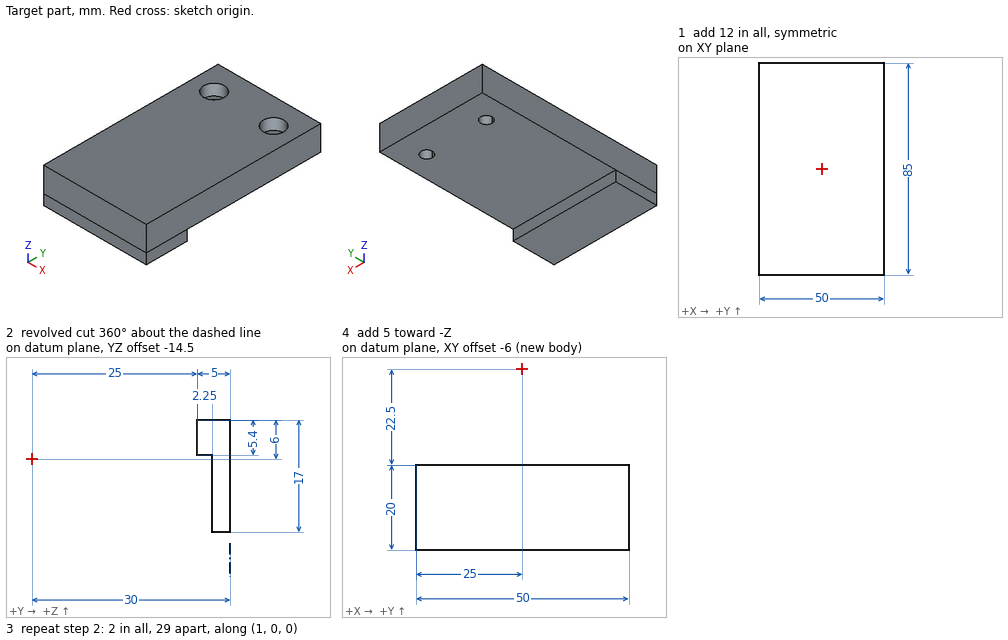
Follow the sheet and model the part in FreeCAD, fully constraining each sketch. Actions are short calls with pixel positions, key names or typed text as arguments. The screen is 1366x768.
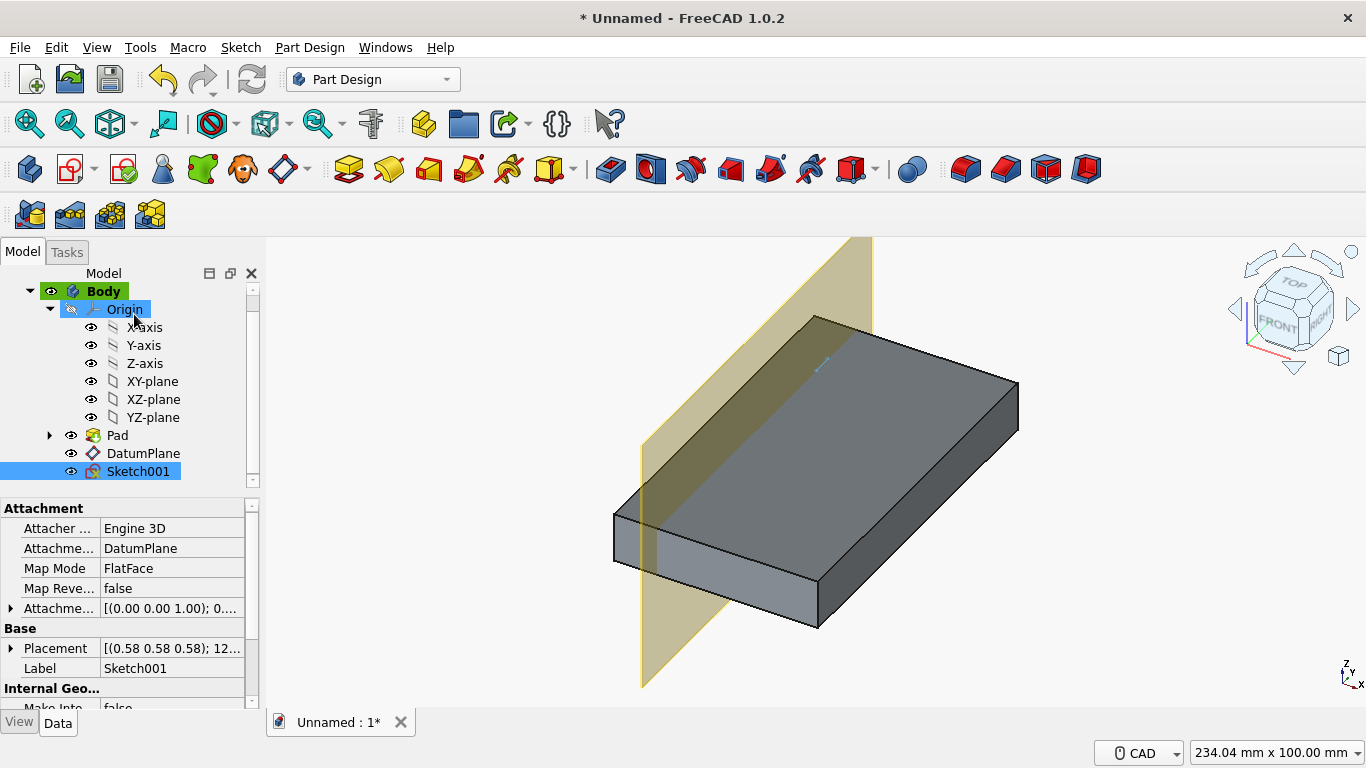
click(692, 170)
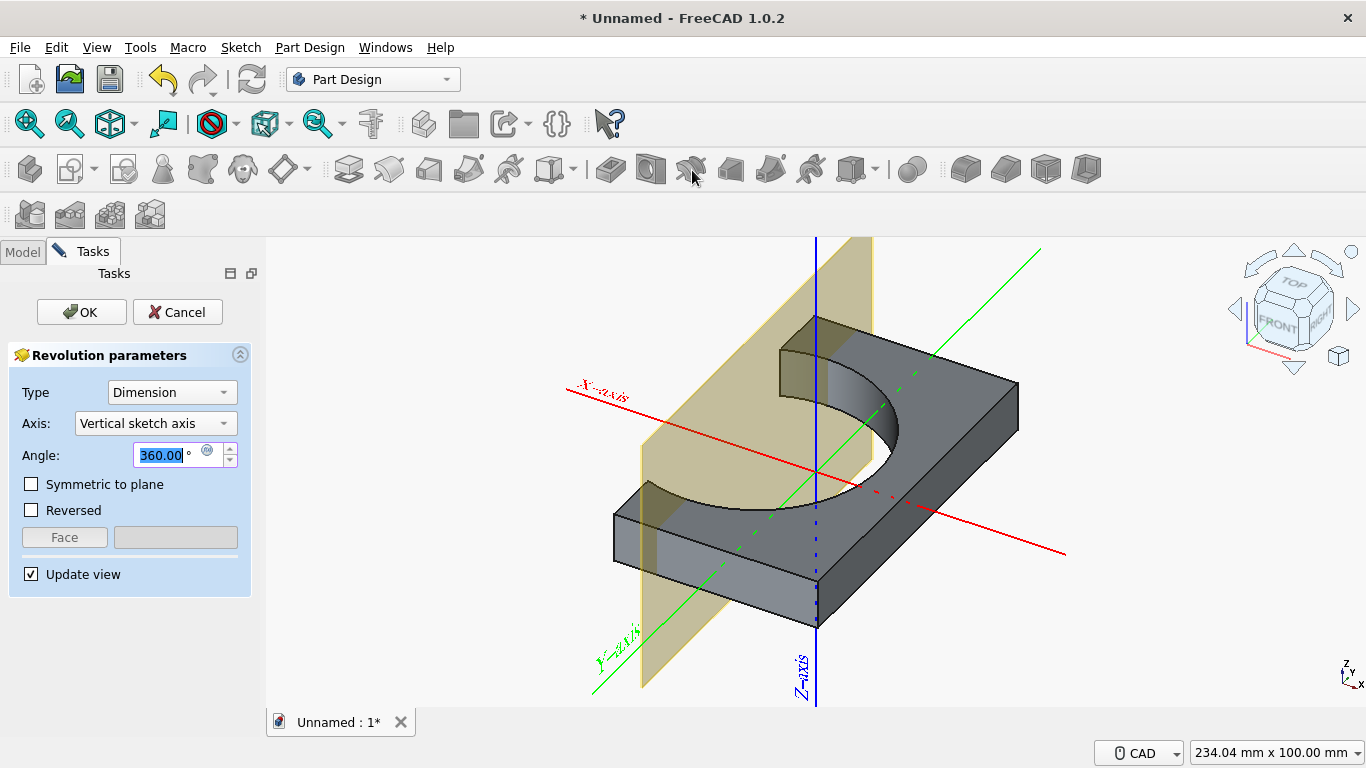
click(156, 424)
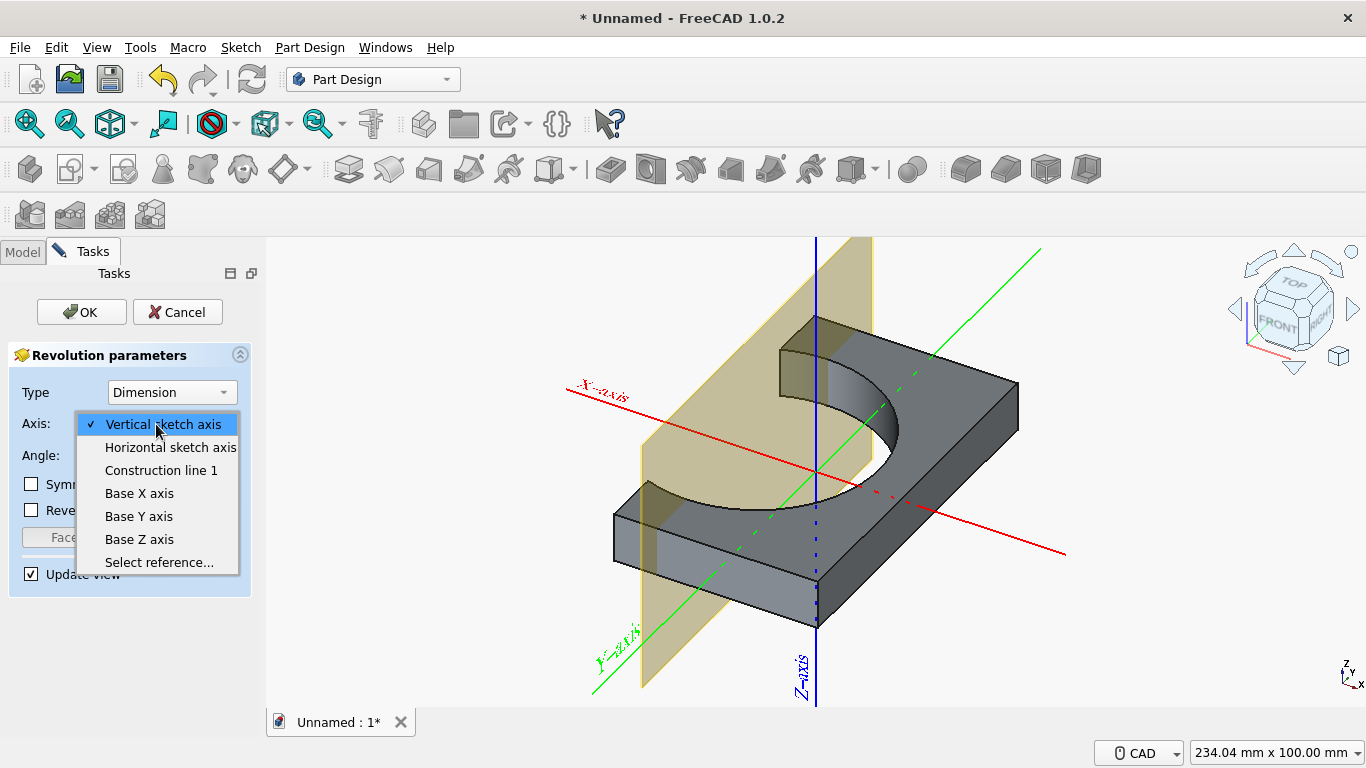
click(156, 470)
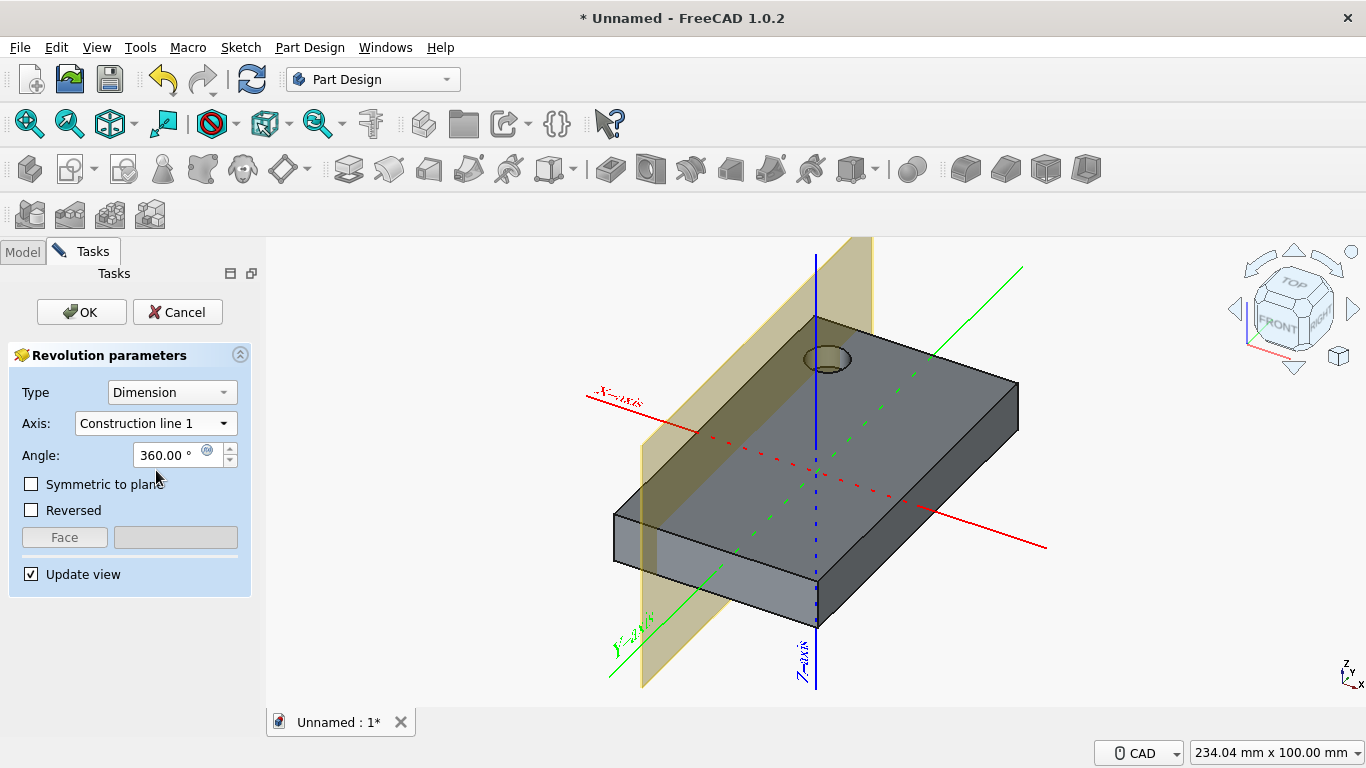
click(82, 312)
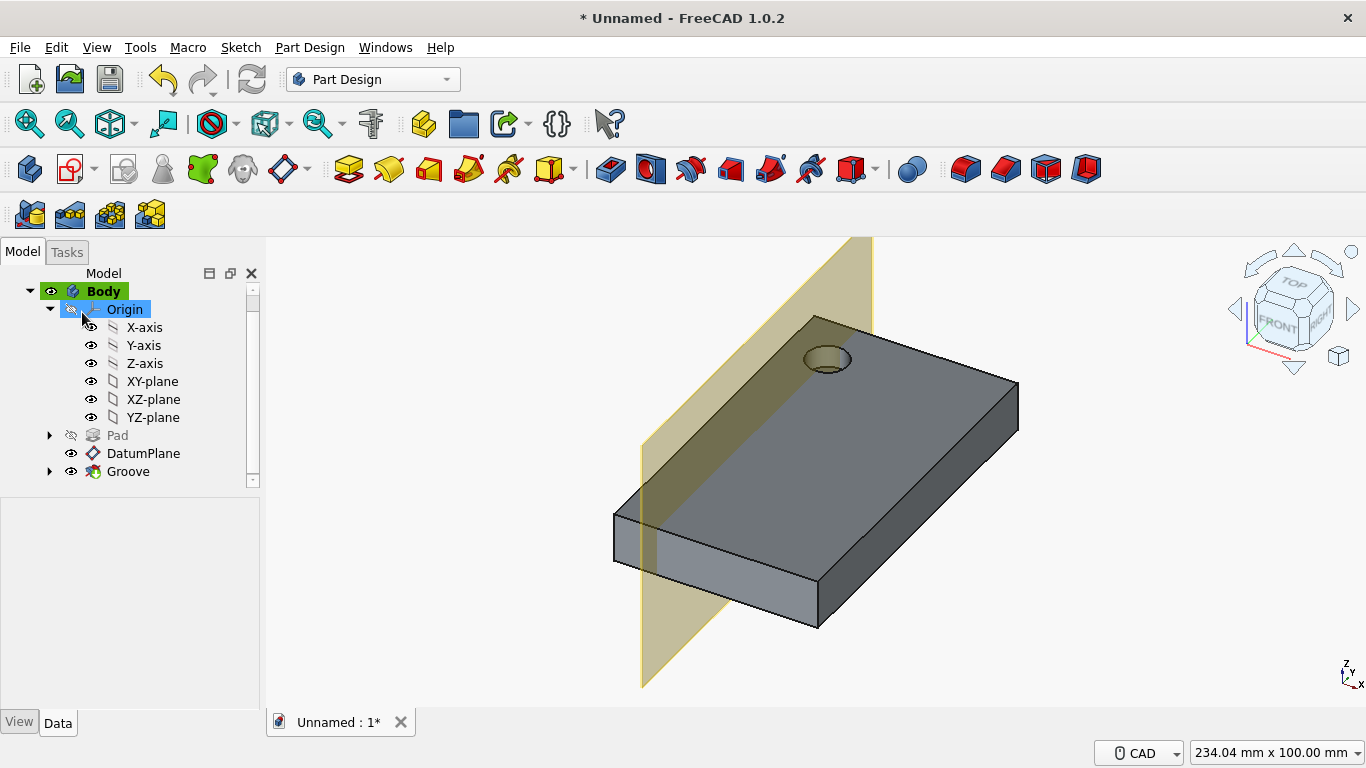
click(116, 453)
key(space)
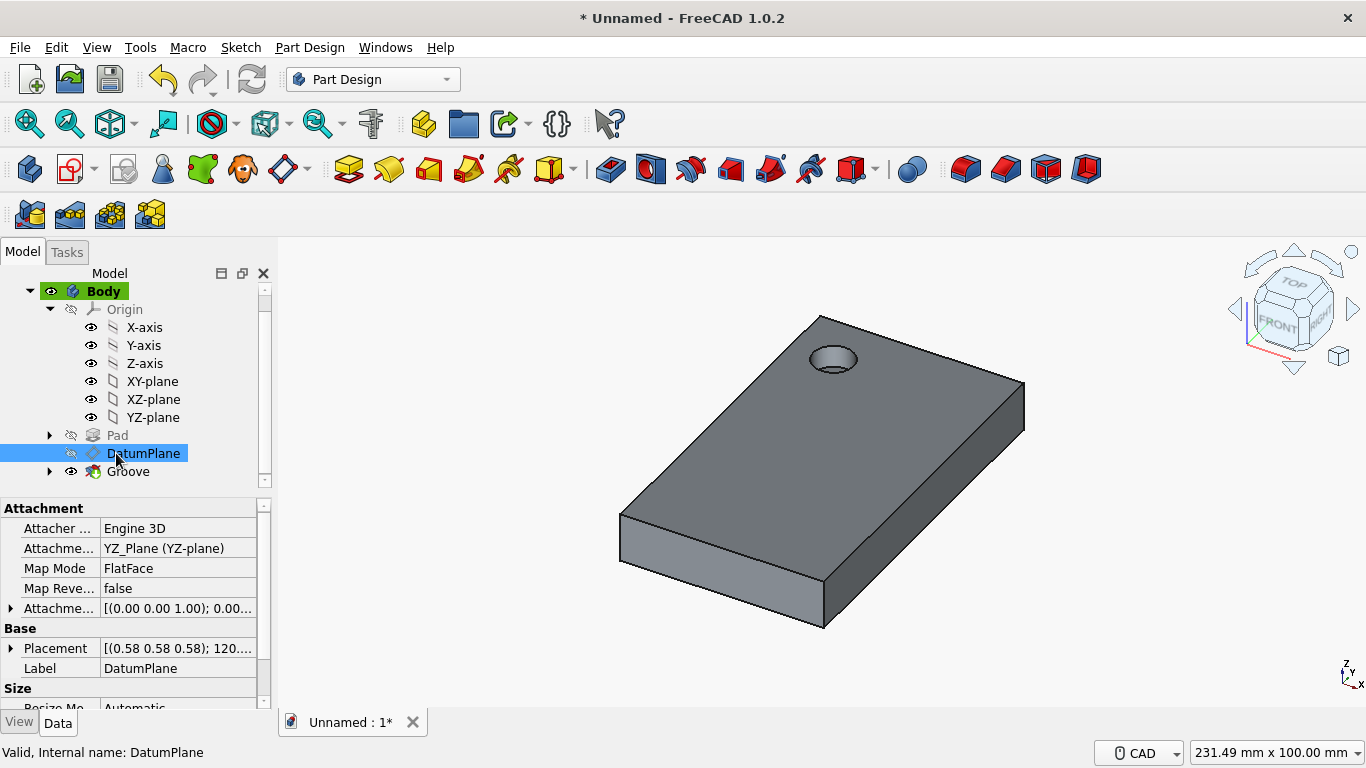
click(116, 471)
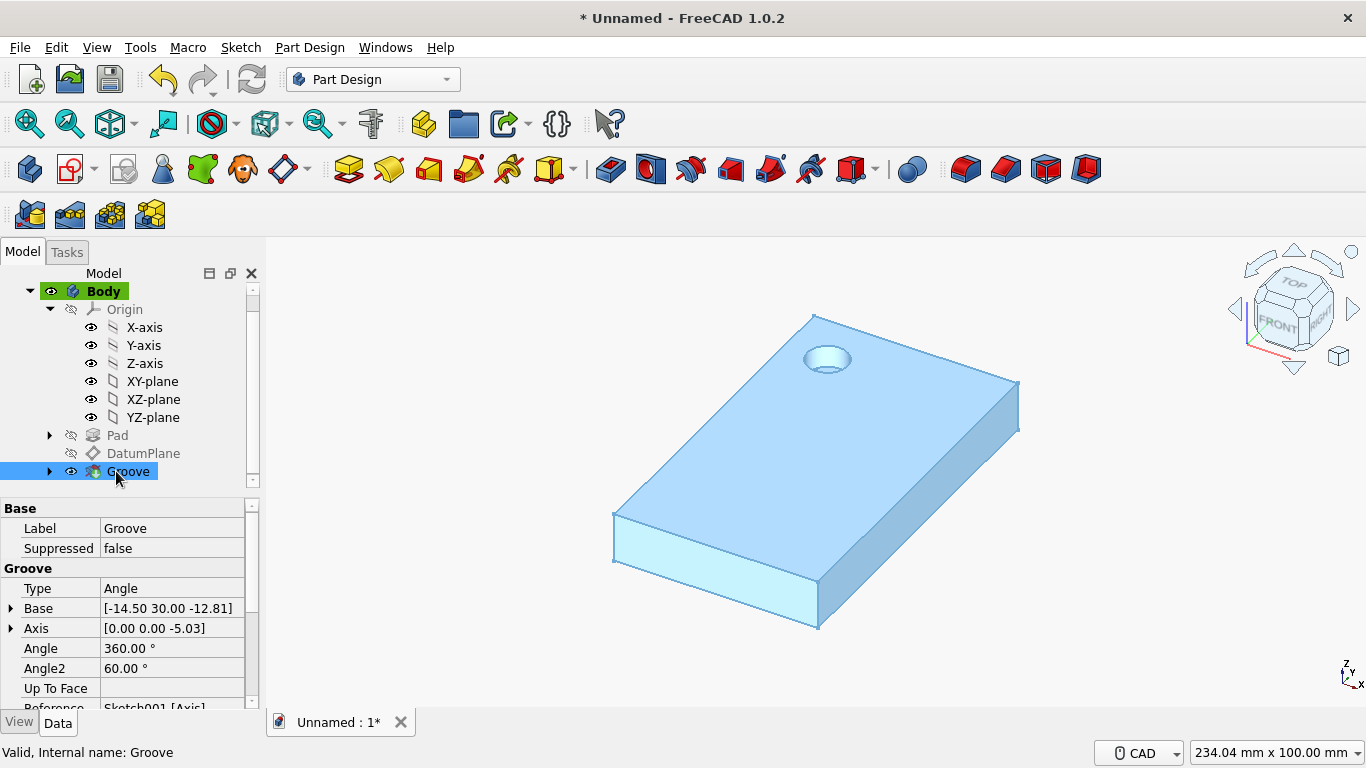
click(70, 214)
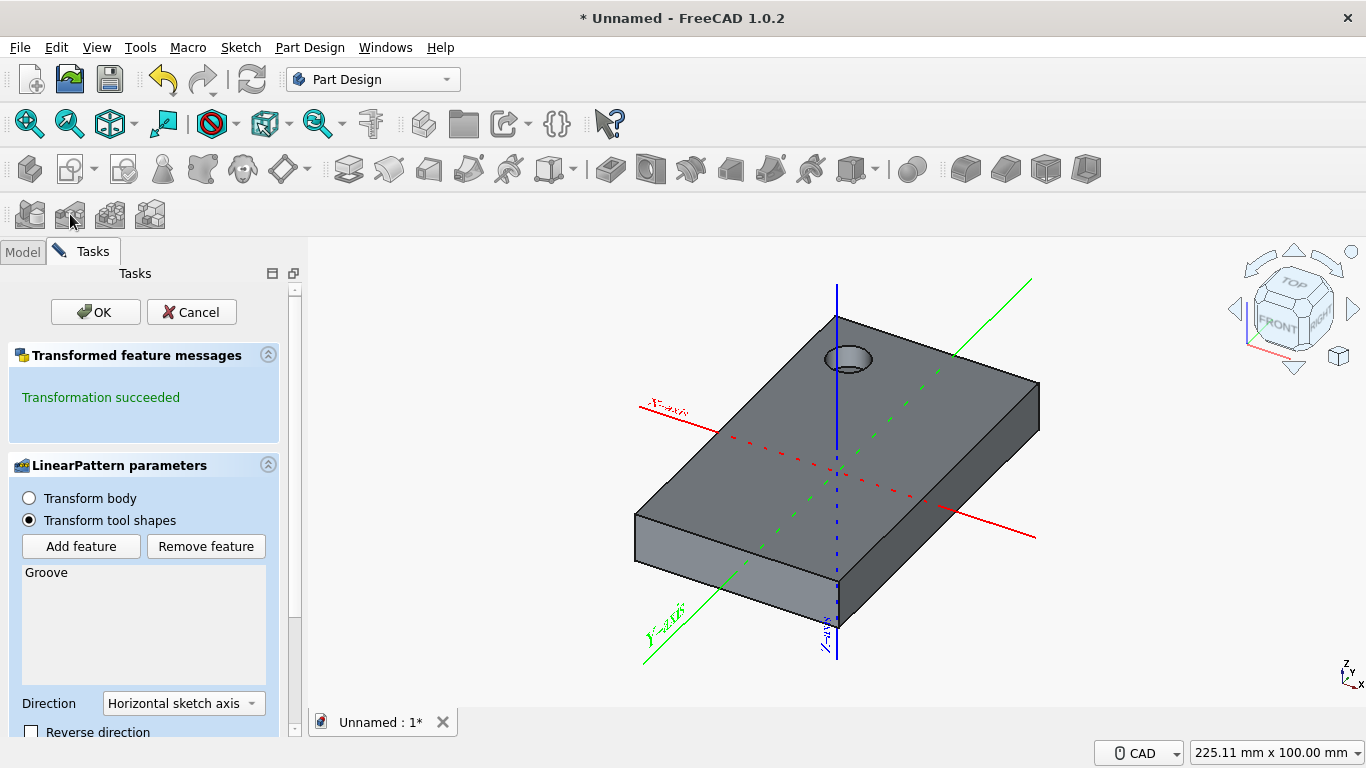
click(184, 704)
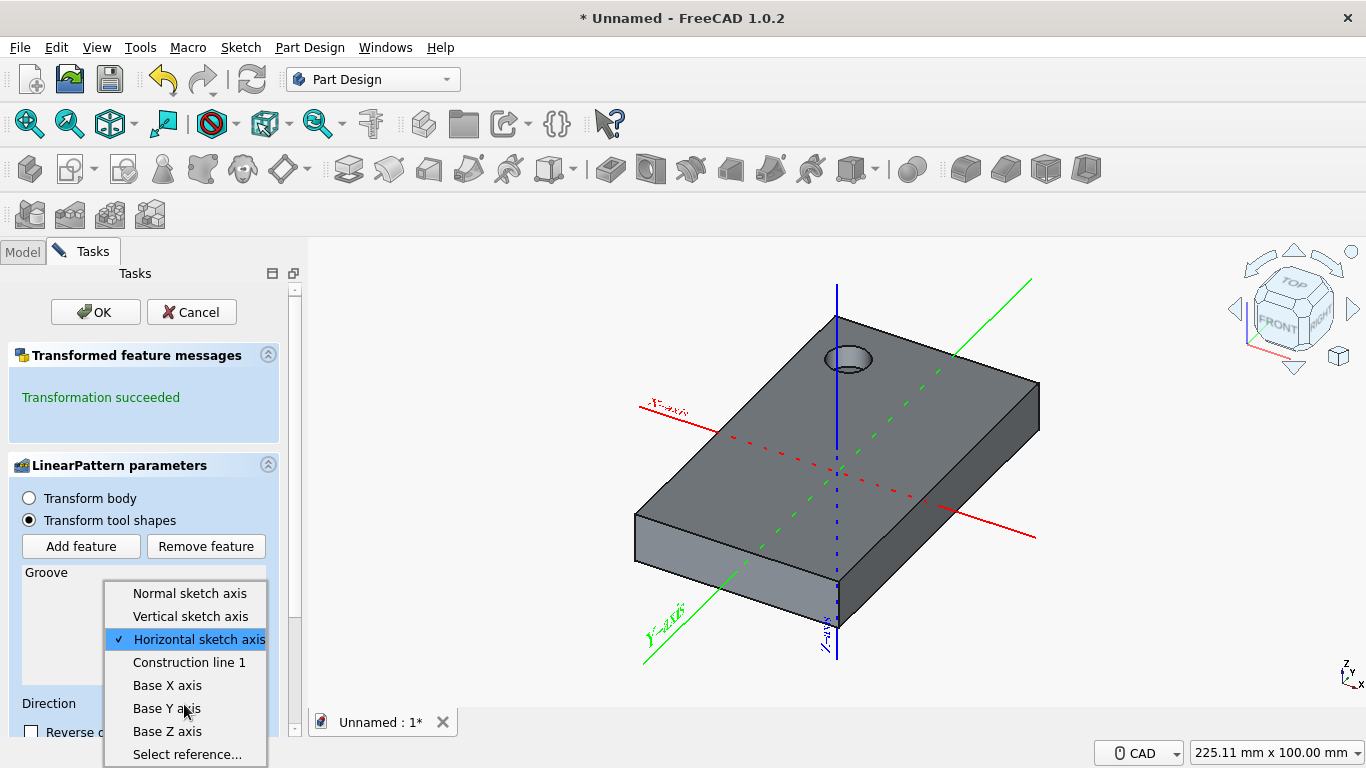
click(184, 686)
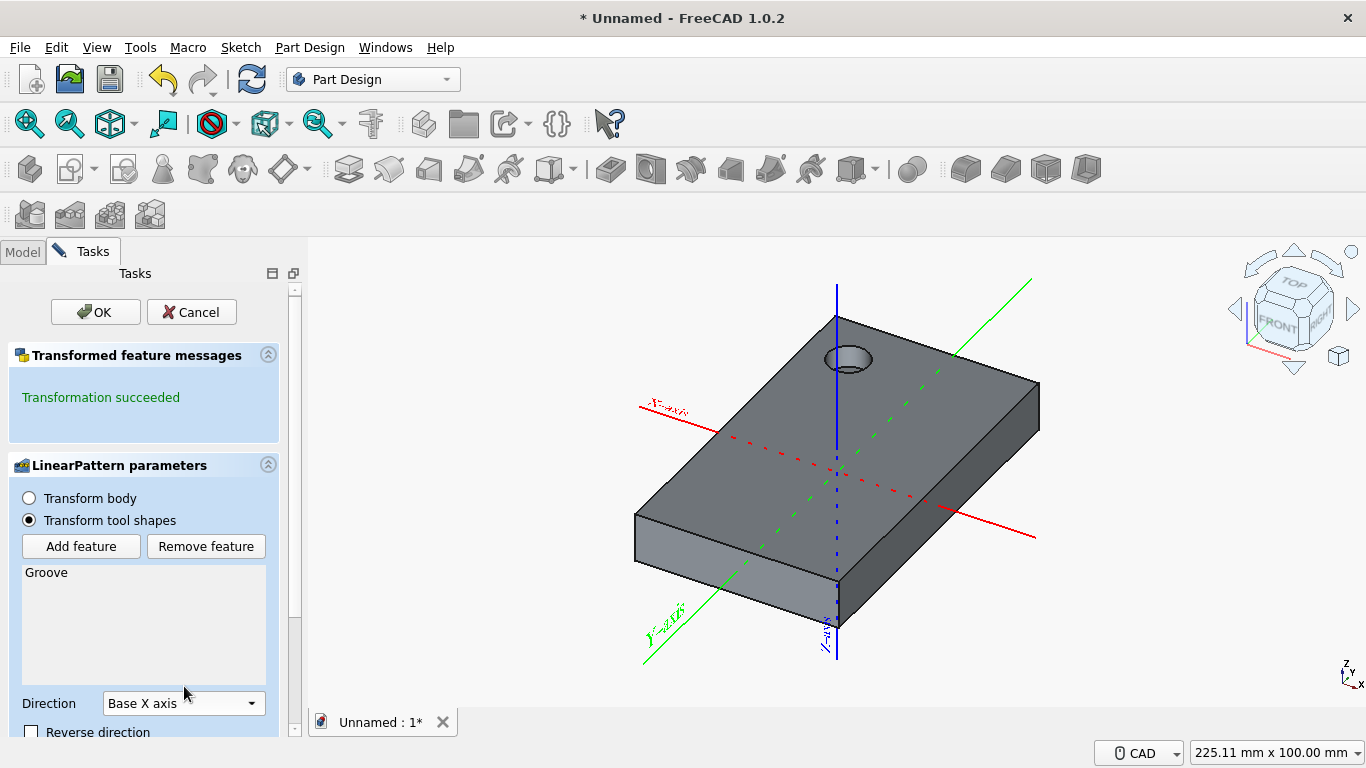
scroll(295, 510, down, 2)